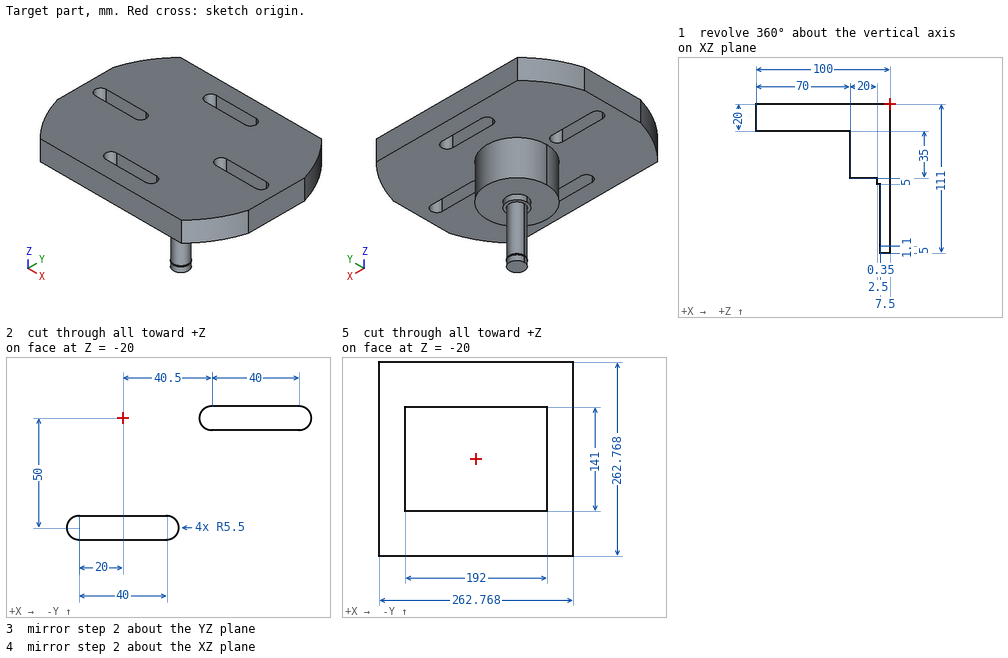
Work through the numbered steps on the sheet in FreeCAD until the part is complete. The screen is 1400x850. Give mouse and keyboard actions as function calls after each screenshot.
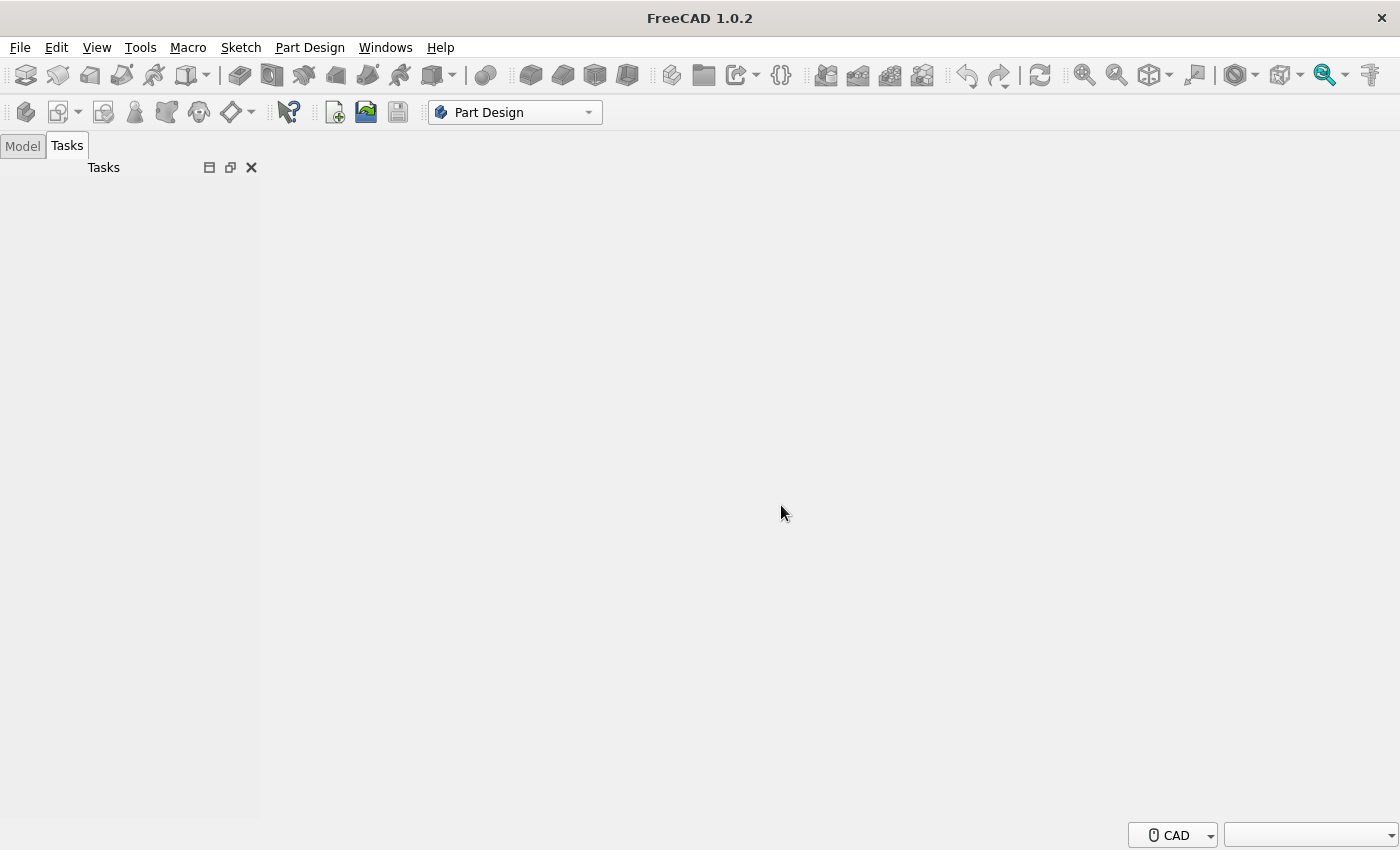
click(334, 112)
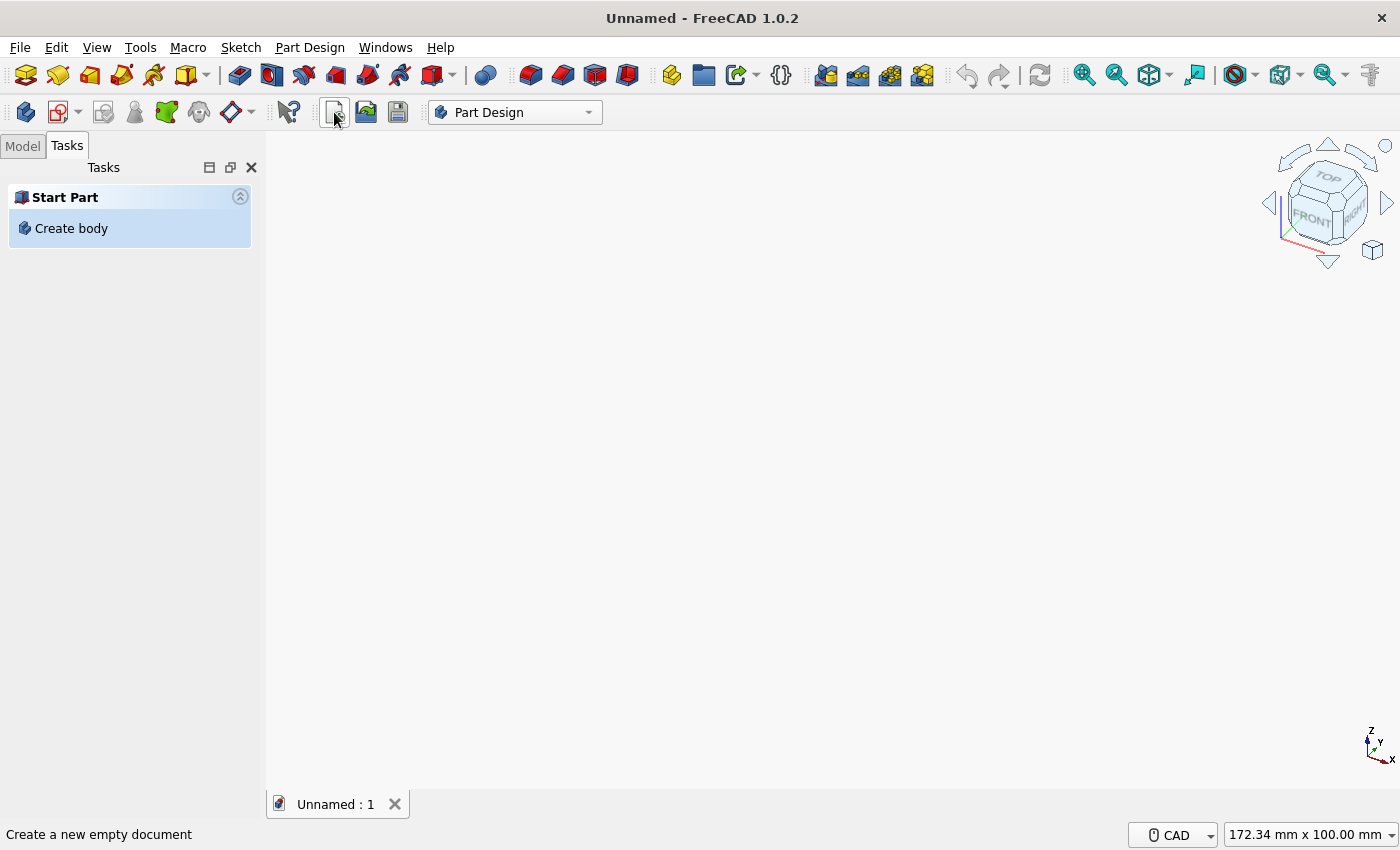
click(58, 112)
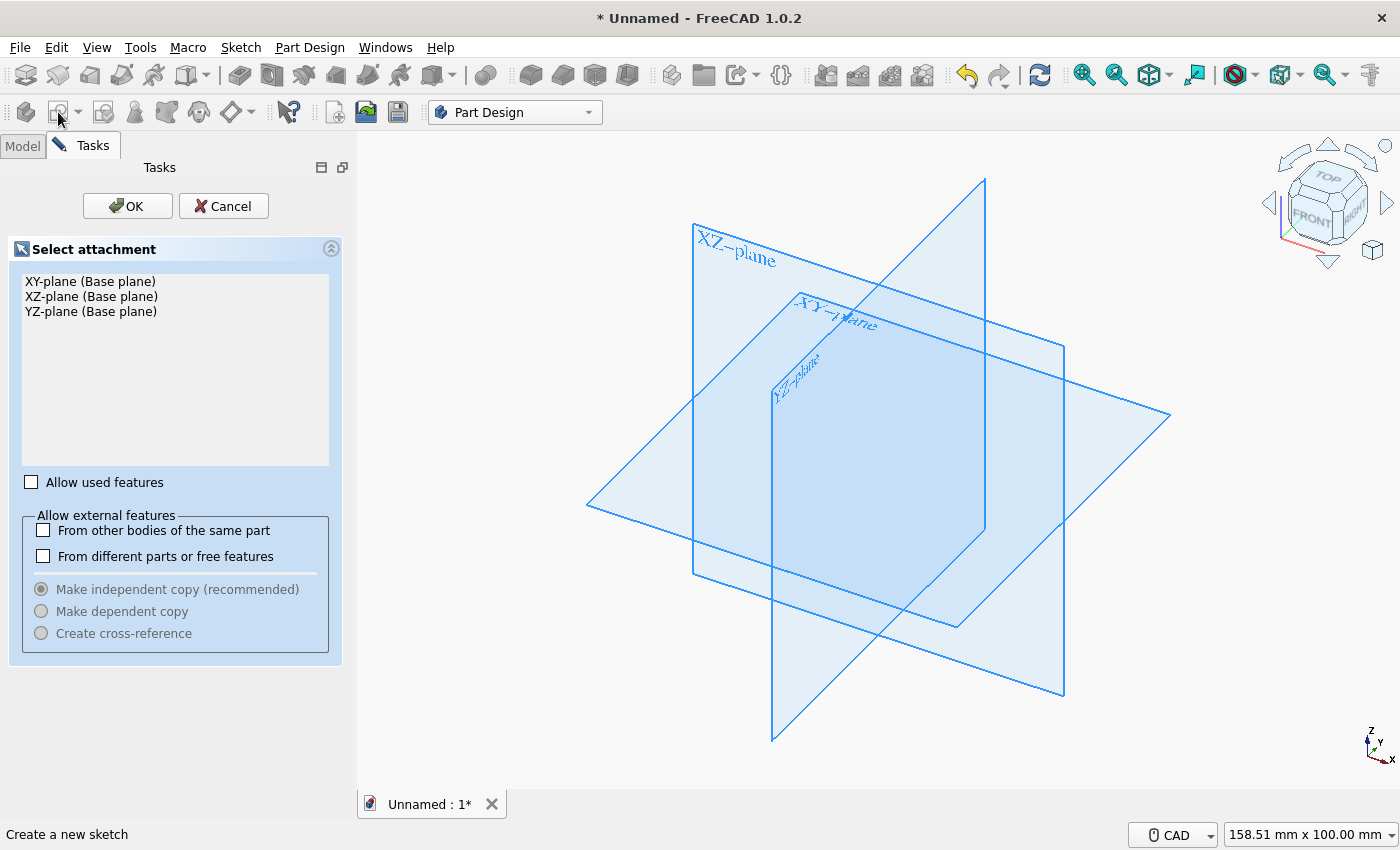
click(82, 296)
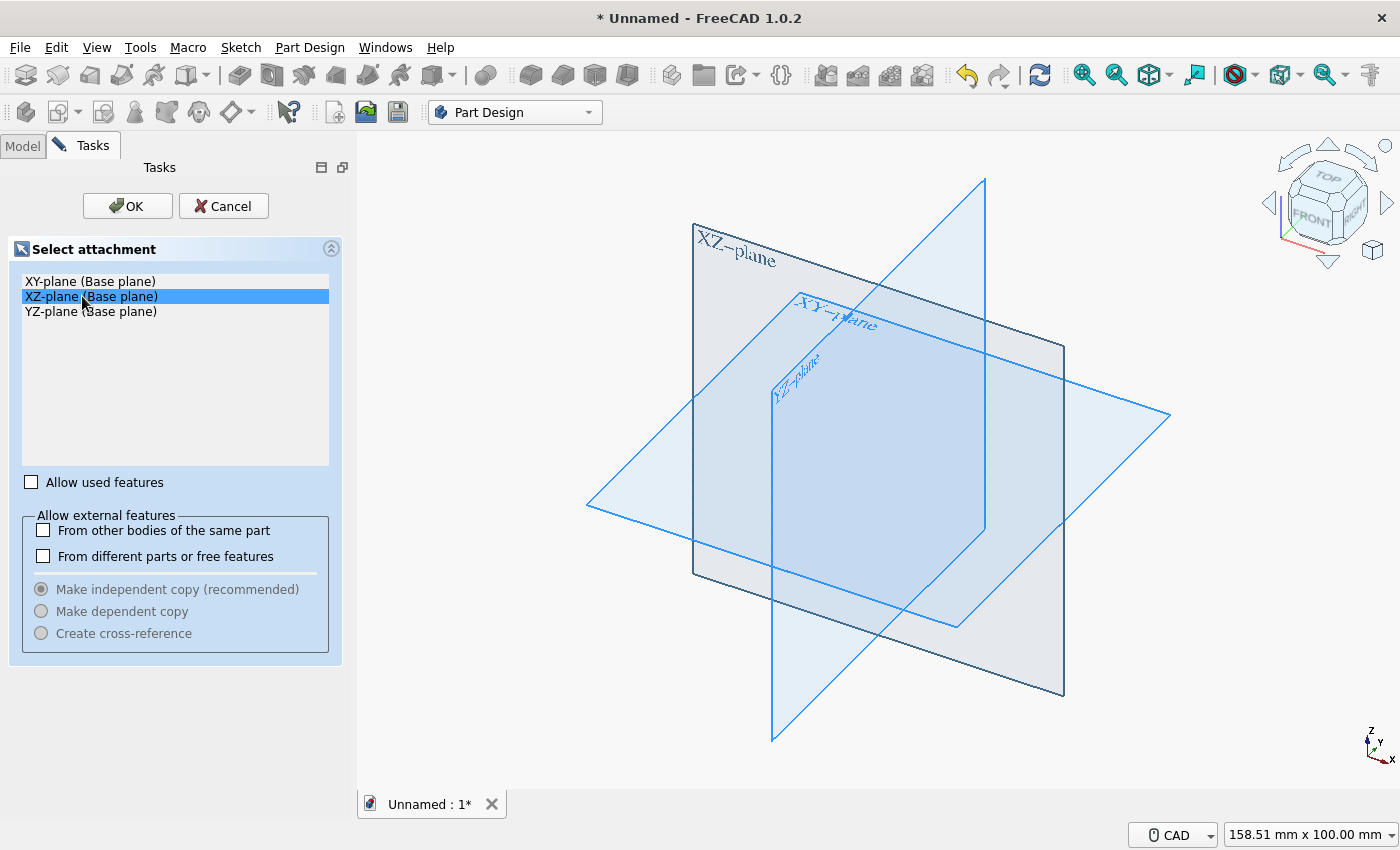
click(128, 206)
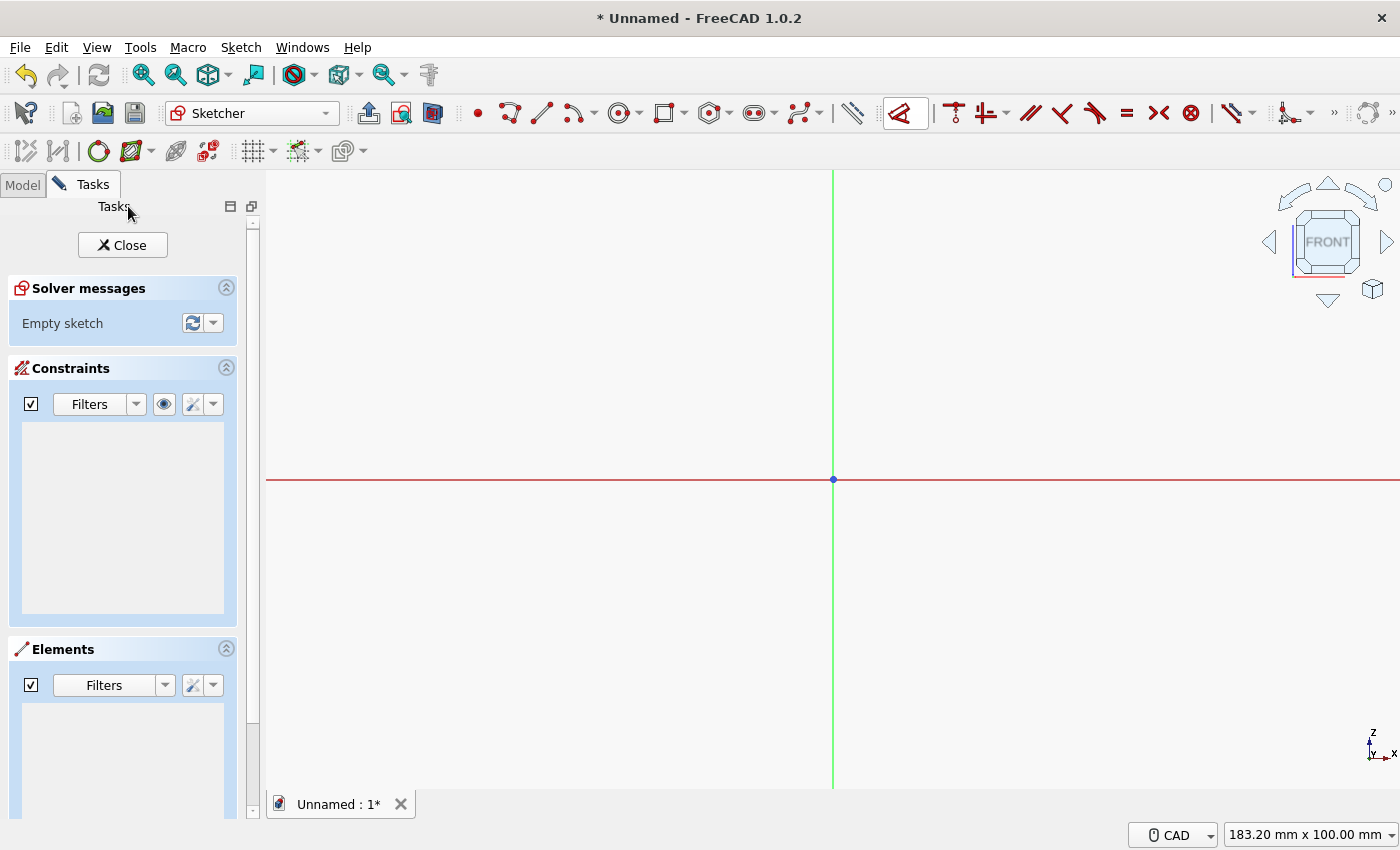
scroll(1058, 198, down, 3)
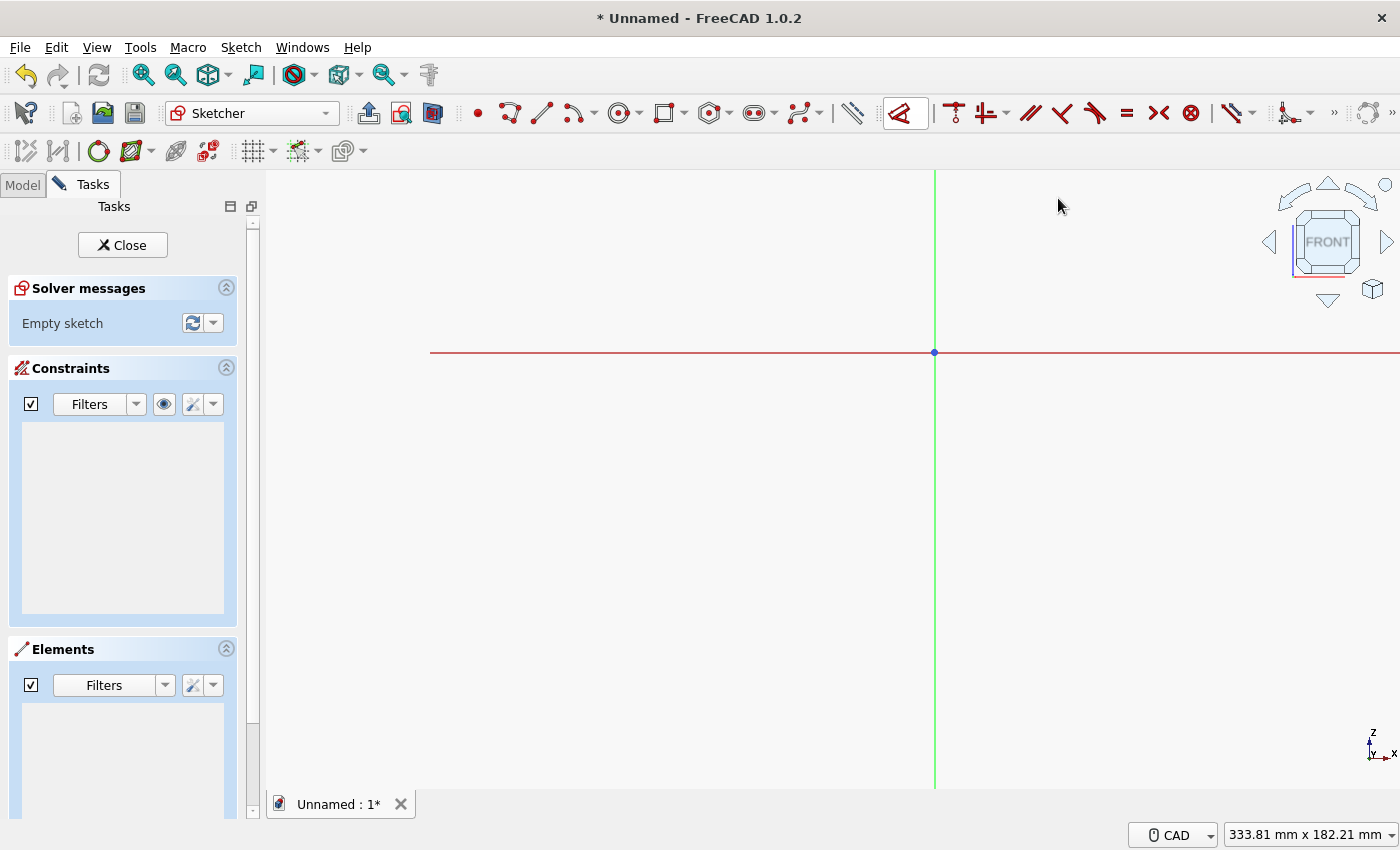
click(510, 114)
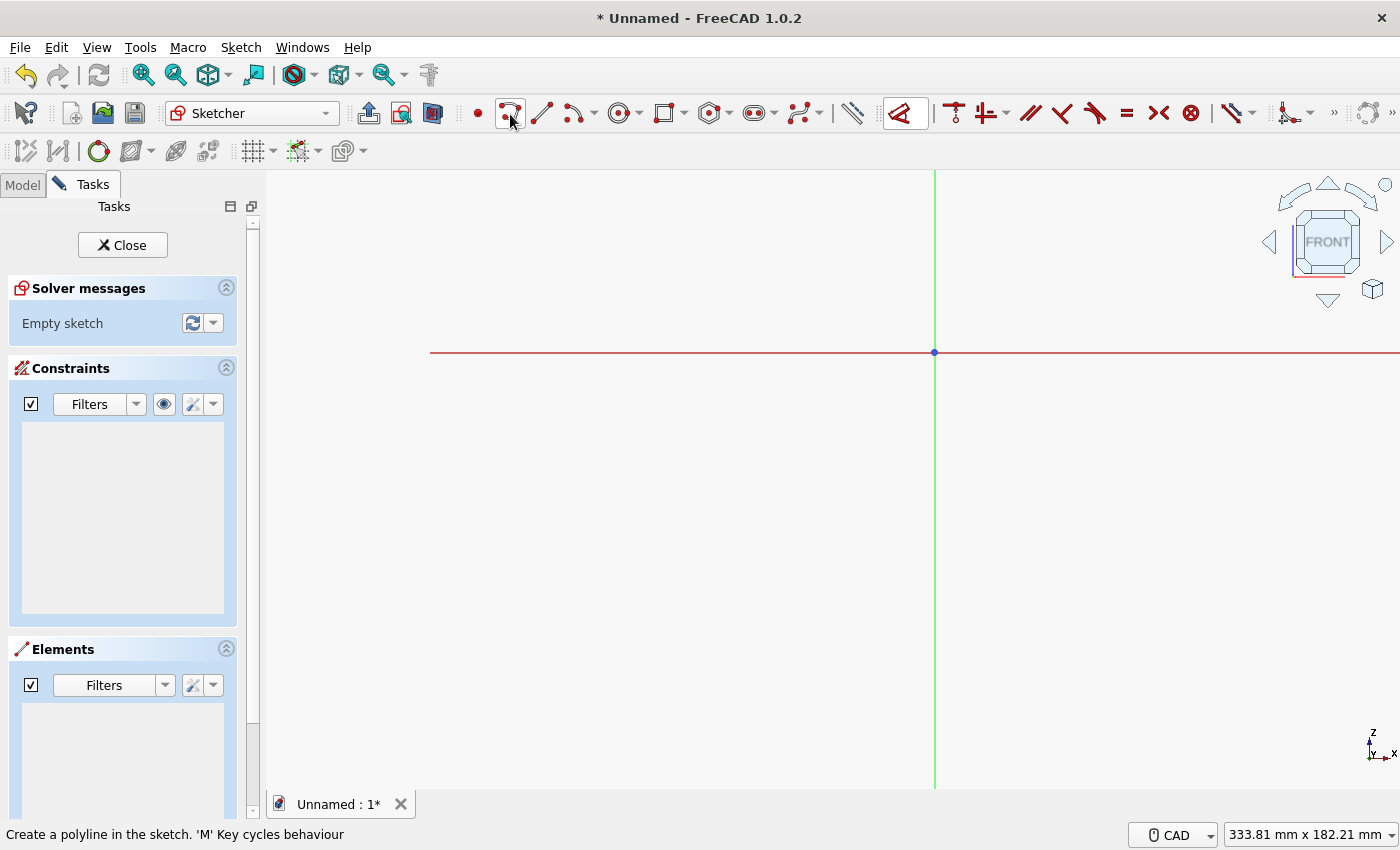
click(935, 353)
click(926, 730)
click(909, 730)
click(909, 713)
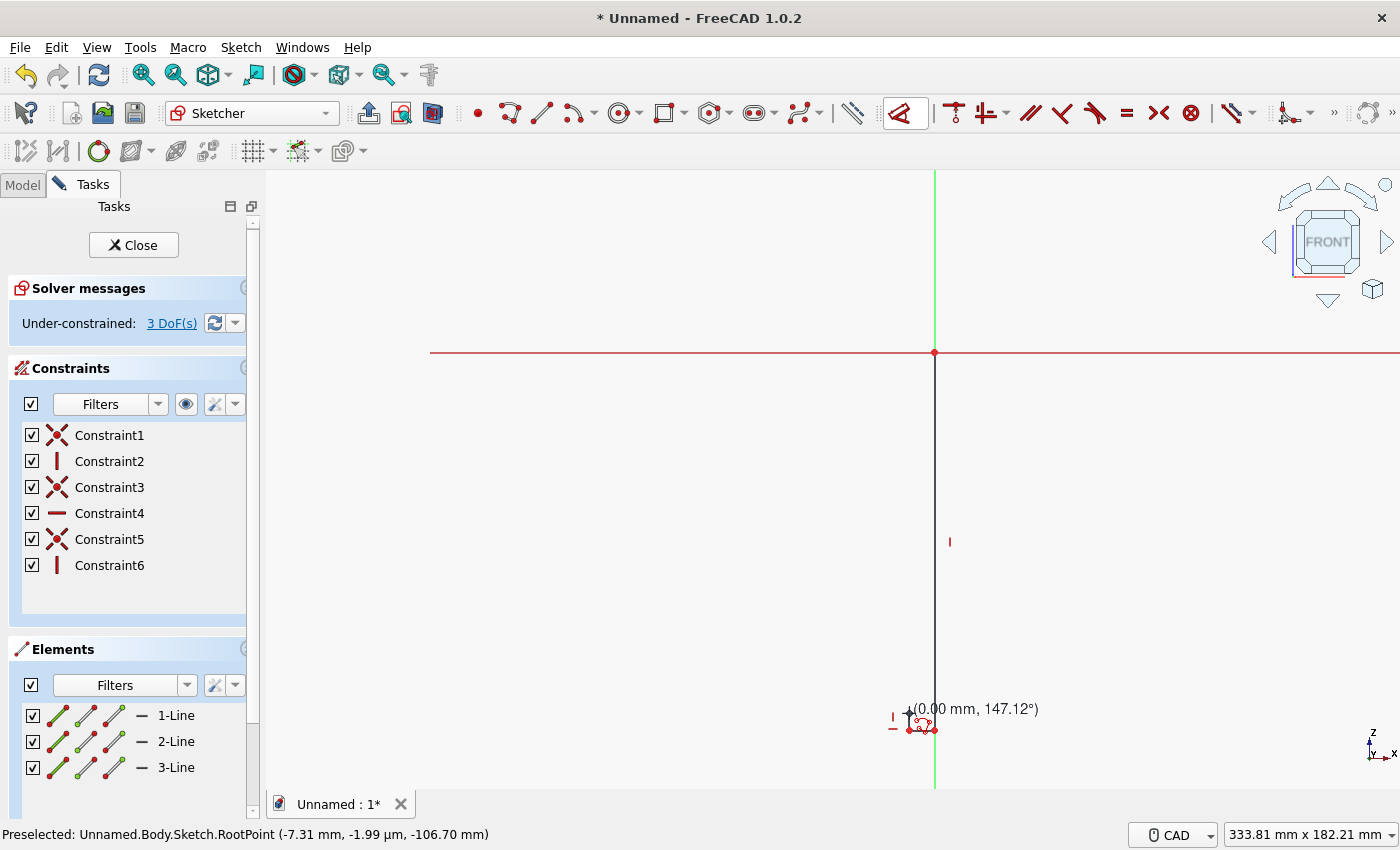
scroll(911, 713, up, 13)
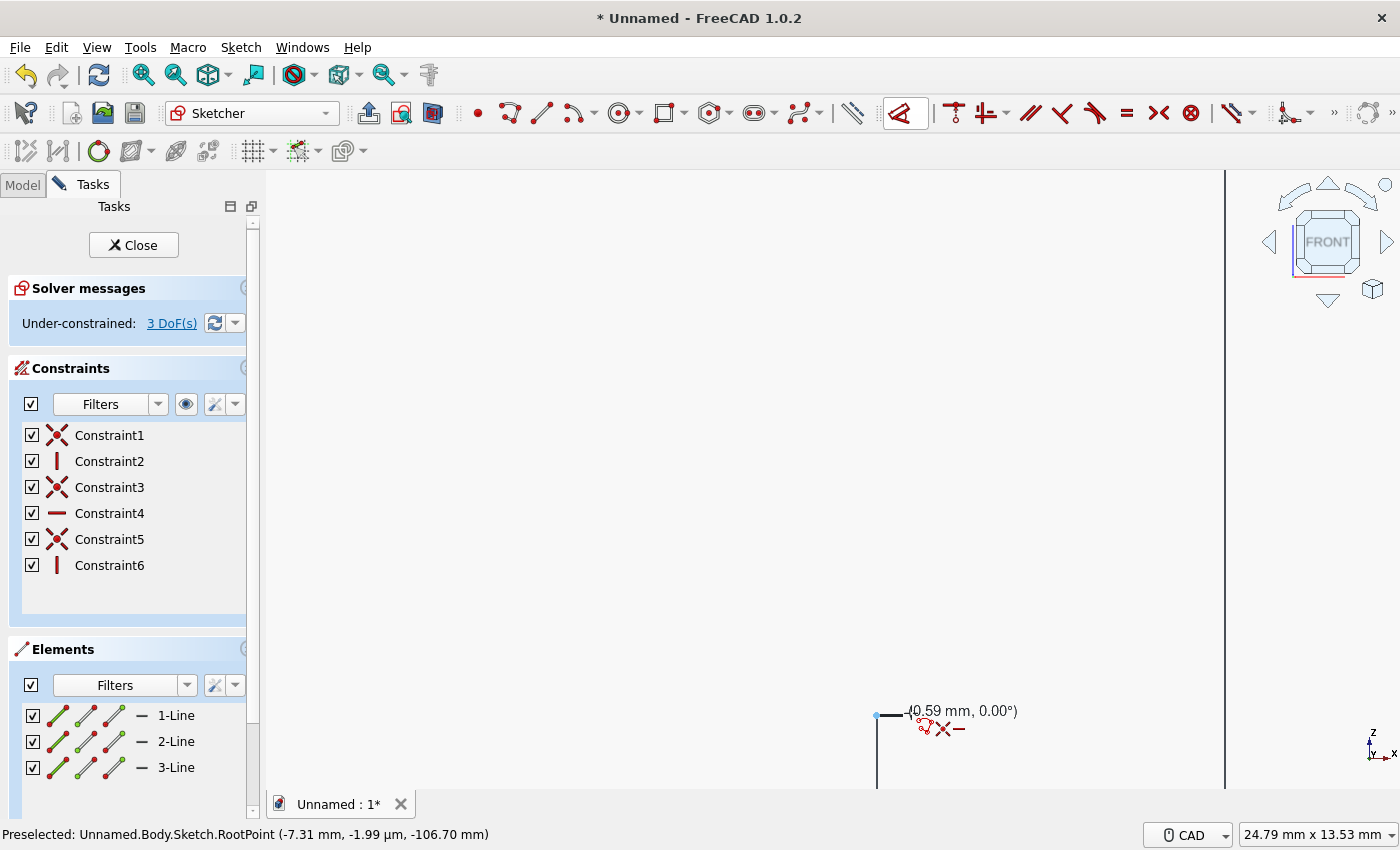
click(898, 702)